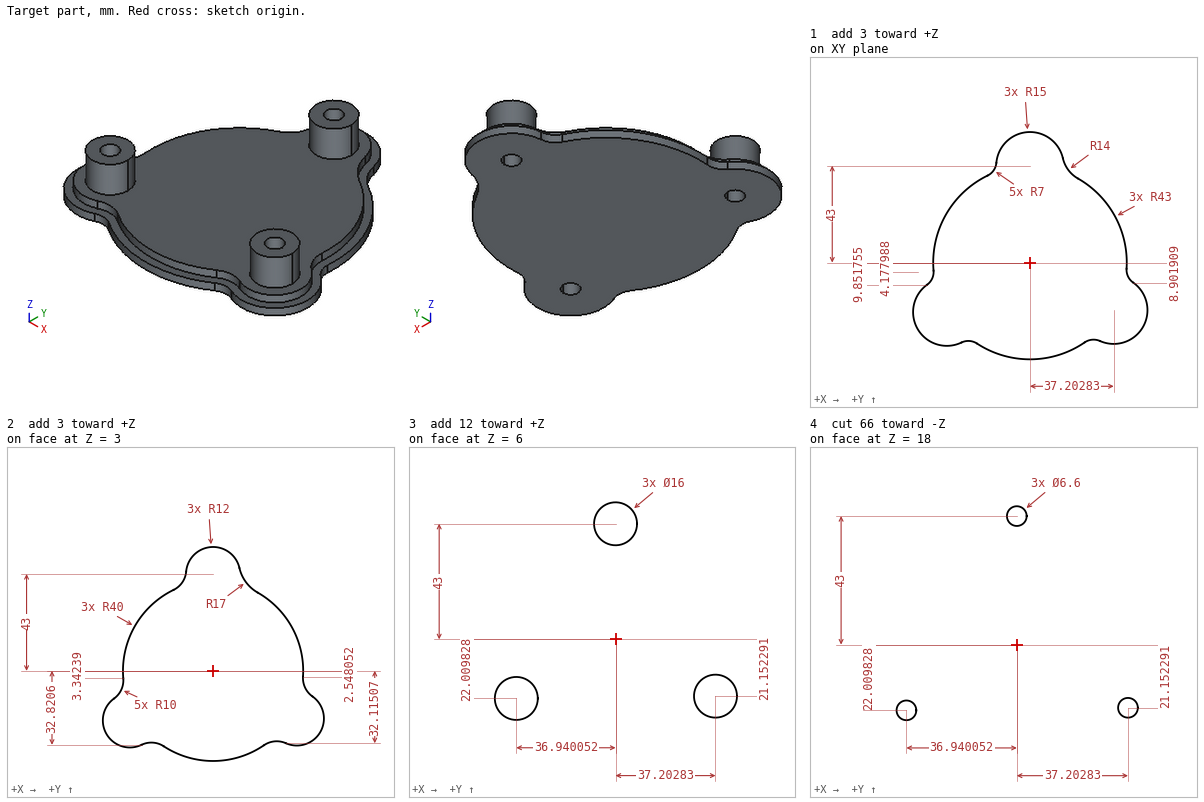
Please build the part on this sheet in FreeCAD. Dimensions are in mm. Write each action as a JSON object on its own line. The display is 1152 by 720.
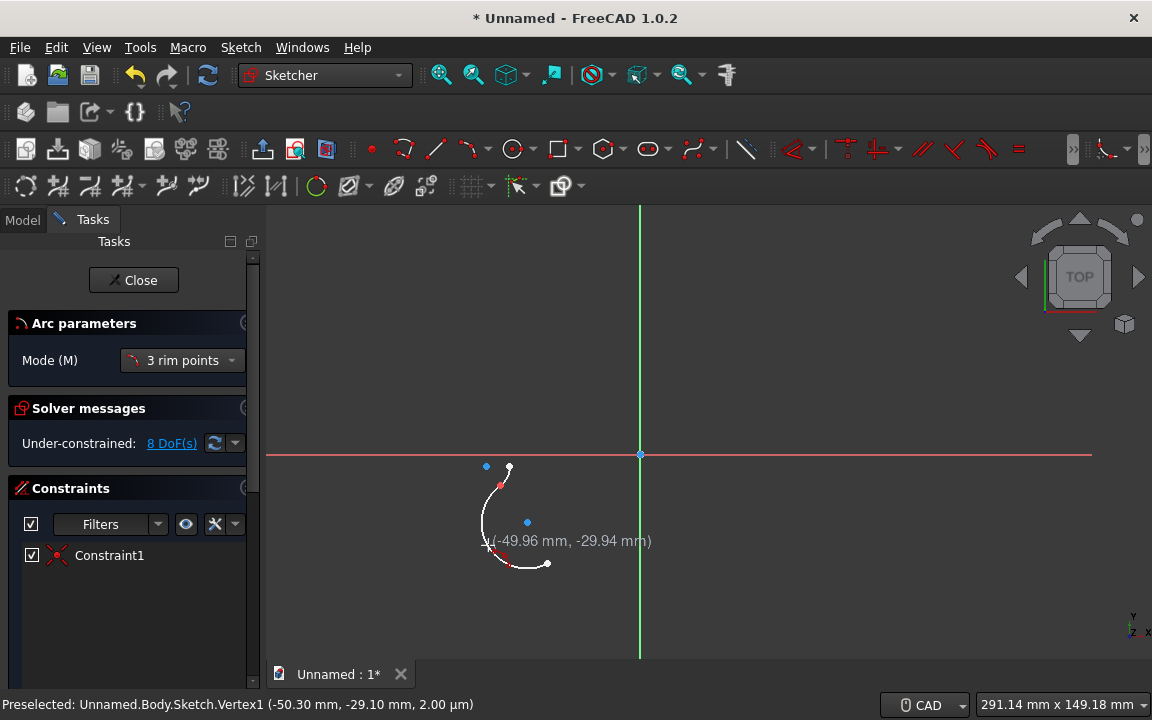
{"action": "left_click", "coordinate": [547, 564]}
{"action": "left_click", "coordinate": [568, 564]}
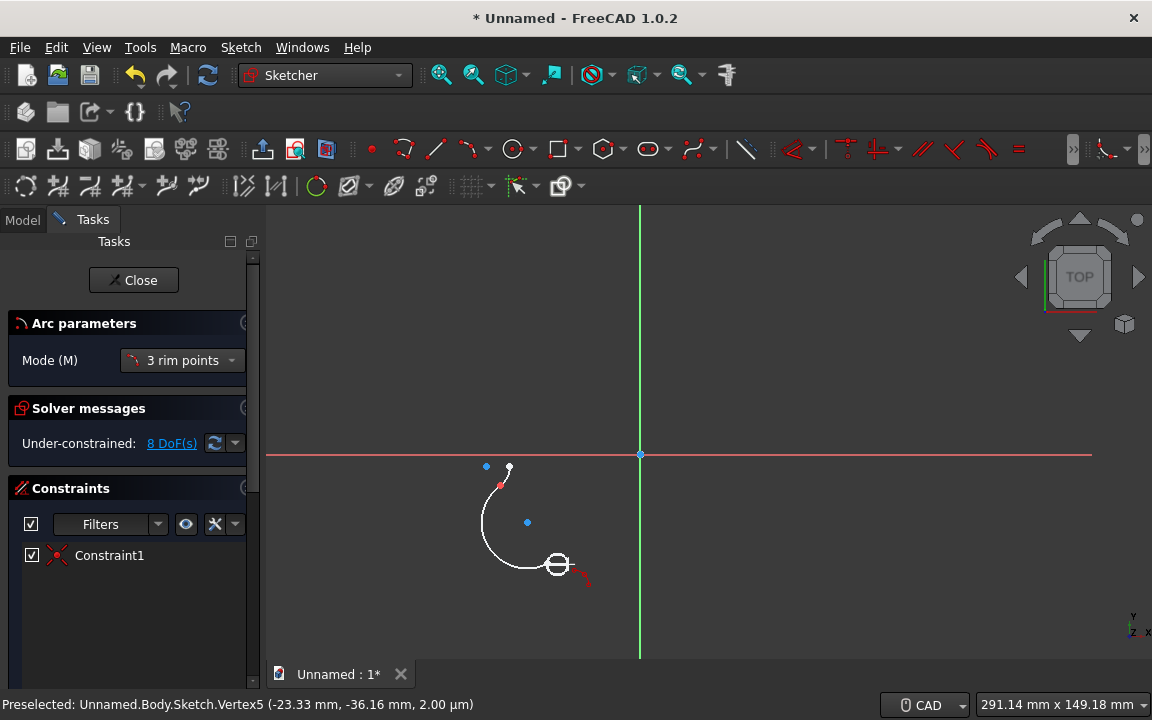
{"action": "scroll", "coordinate": [558, 561], "scroll_direction": "up", "scroll_amount": 9}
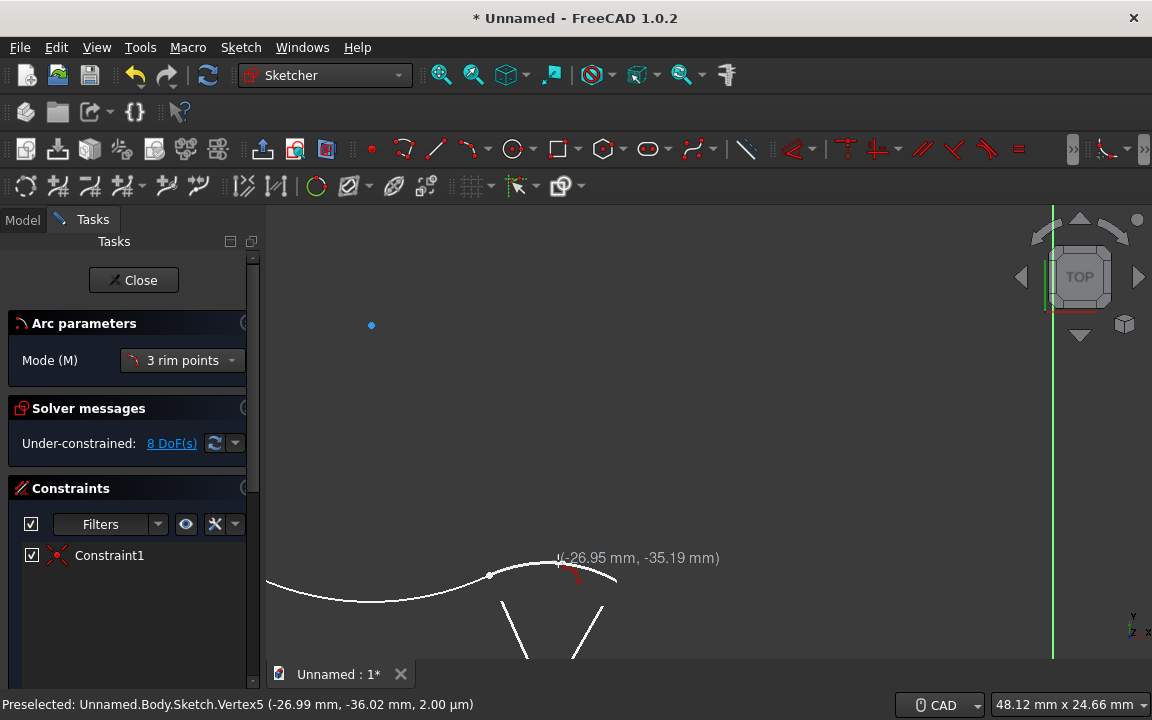
{"action": "left_click", "coordinate": [557, 557]}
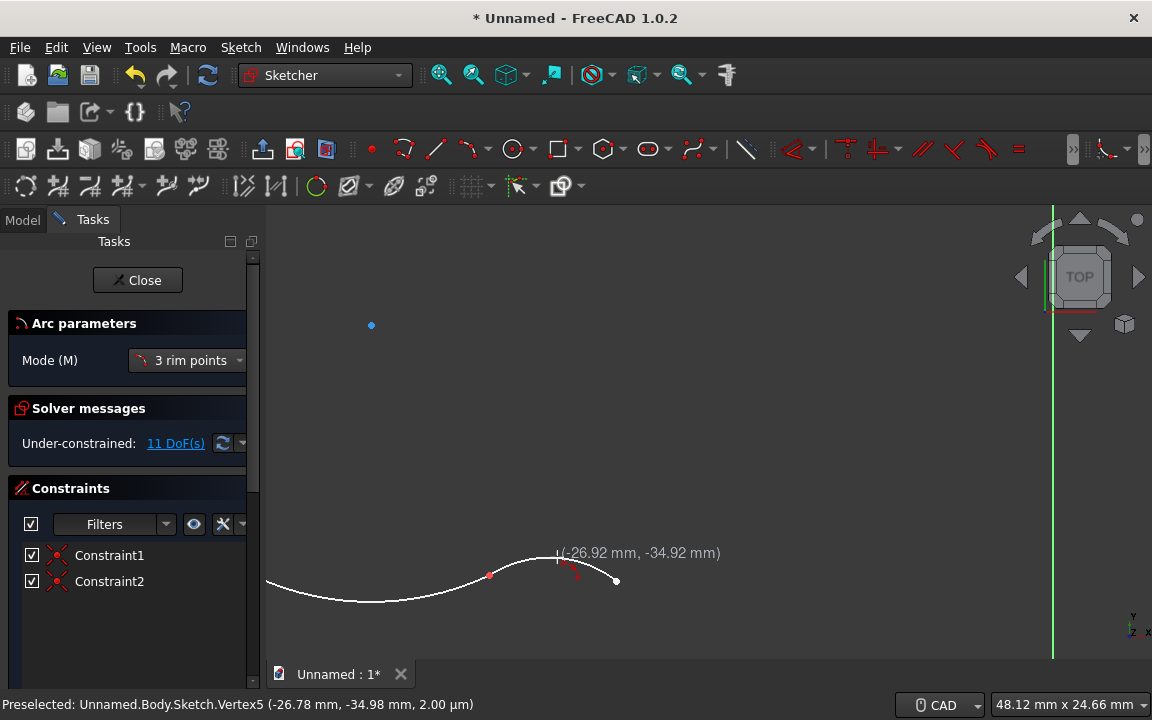
{"action": "scroll", "coordinate": [558, 562], "scroll_direction": "down", "scroll_amount": 9}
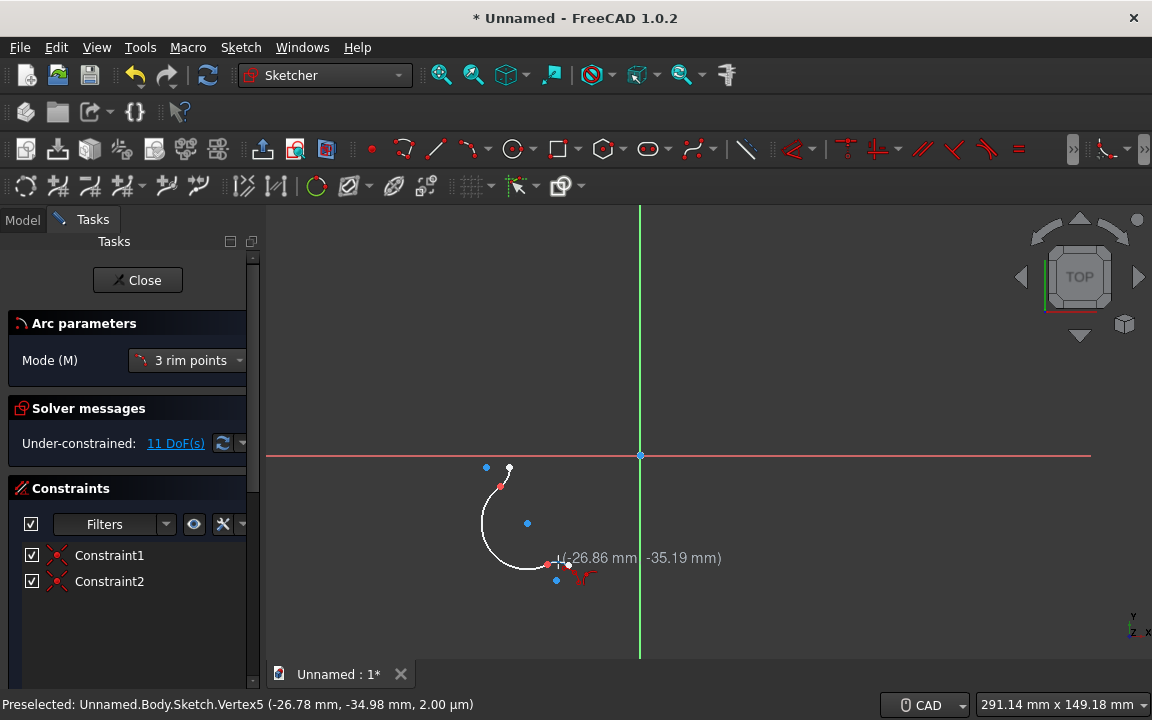
{"action": "left_click", "coordinate": [568, 566]}
{"action": "left_click", "coordinate": [714, 564]}
{"action": "left_click", "coordinate": [626, 586]}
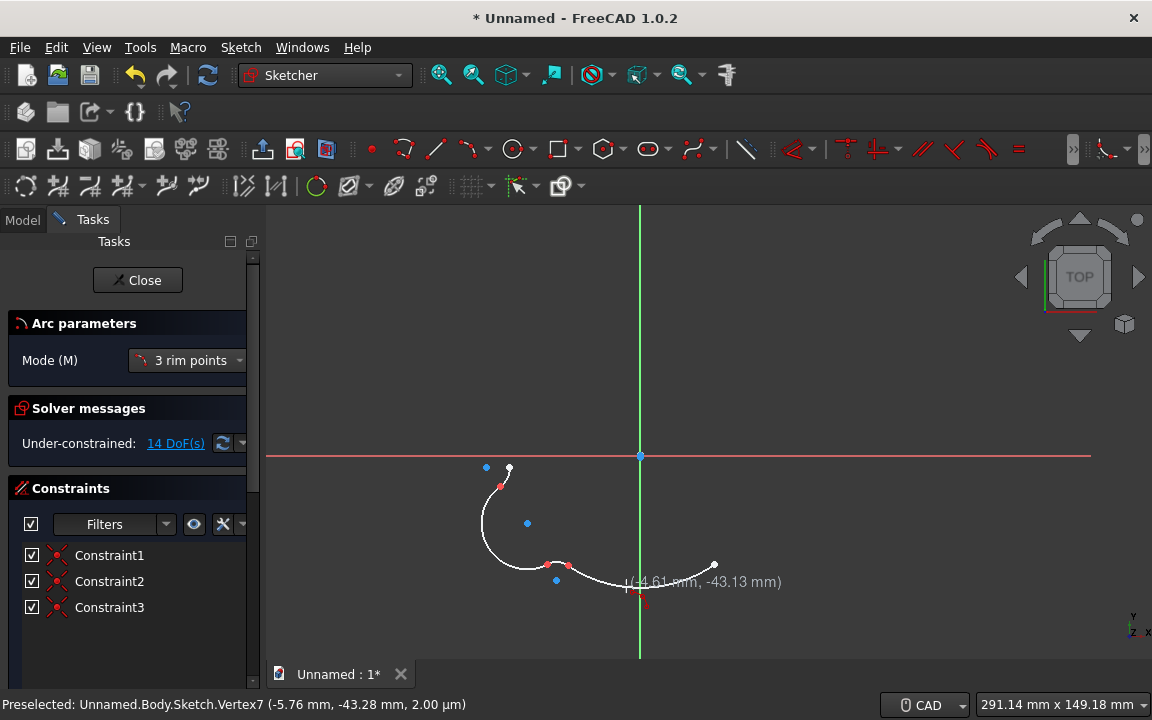
{"action": "left_click", "coordinate": [714, 565]}
{"action": "left_click", "coordinate": [735, 562]}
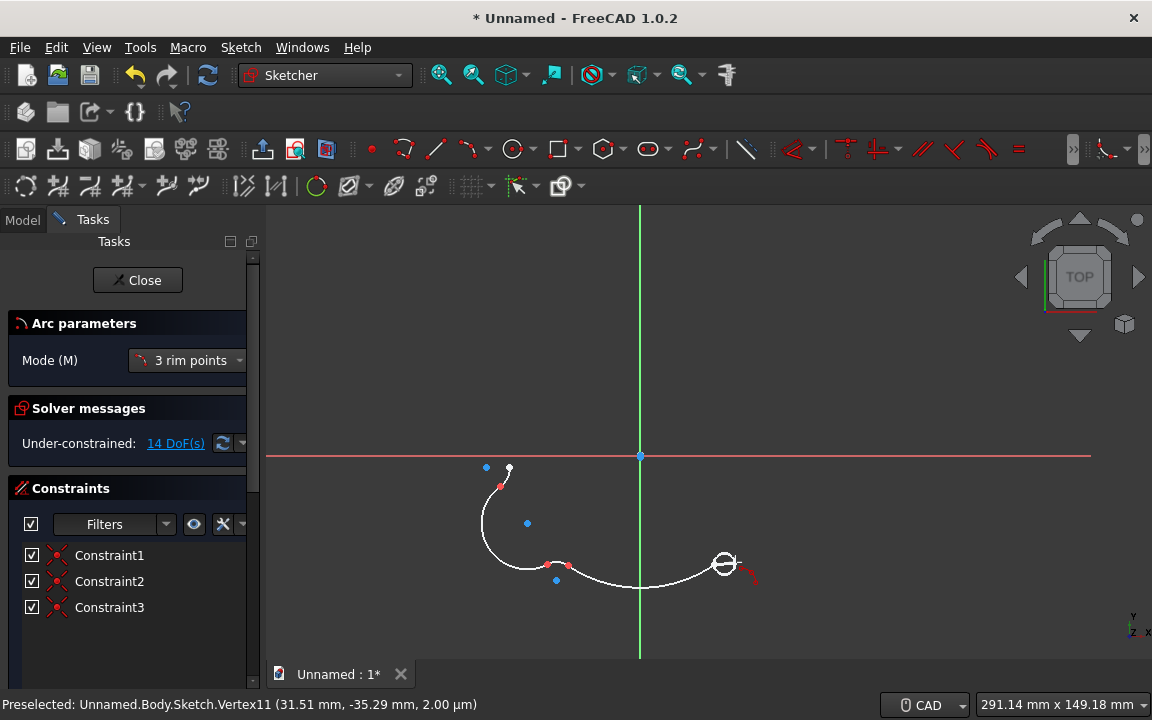
{"action": "scroll", "coordinate": [724, 560], "scroll_direction": "up", "scroll_amount": 9}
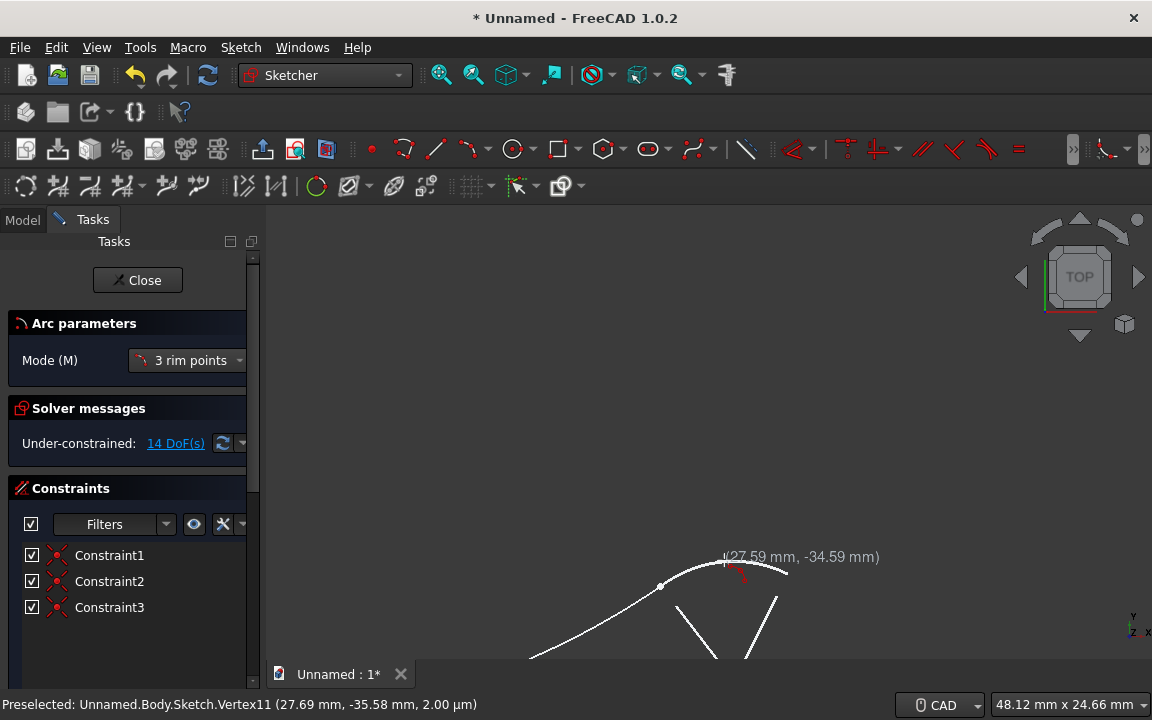
{"action": "left_click", "coordinate": [722, 556]}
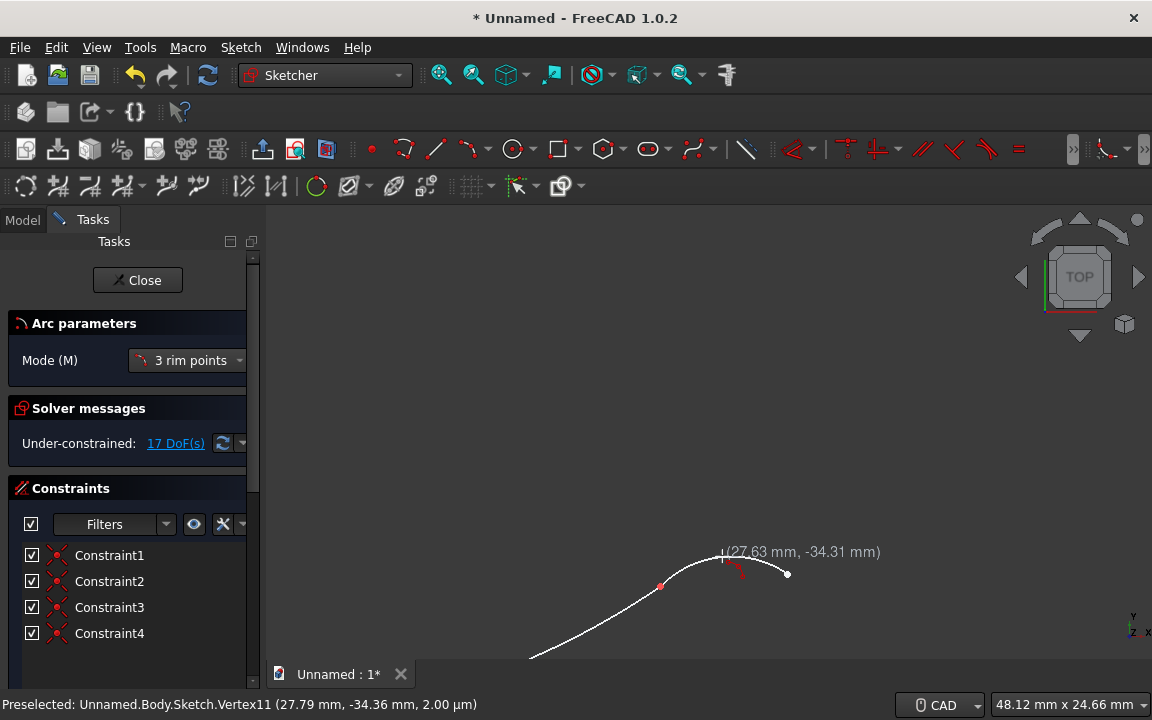
{"action": "scroll", "coordinate": [724, 560], "scroll_direction": "down", "scroll_amount": 9}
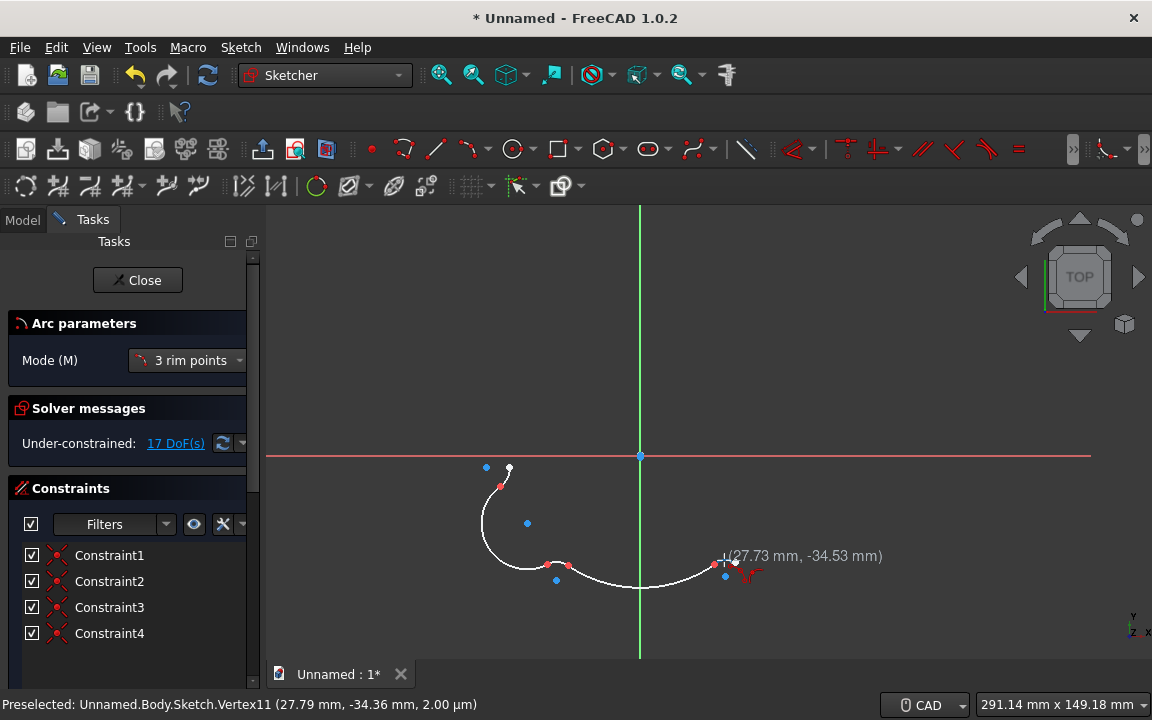
{"action": "left_click", "coordinate": [735, 563]}
{"action": "left_click", "coordinate": [780, 483]}
{"action": "left_click", "coordinate": [793, 543]}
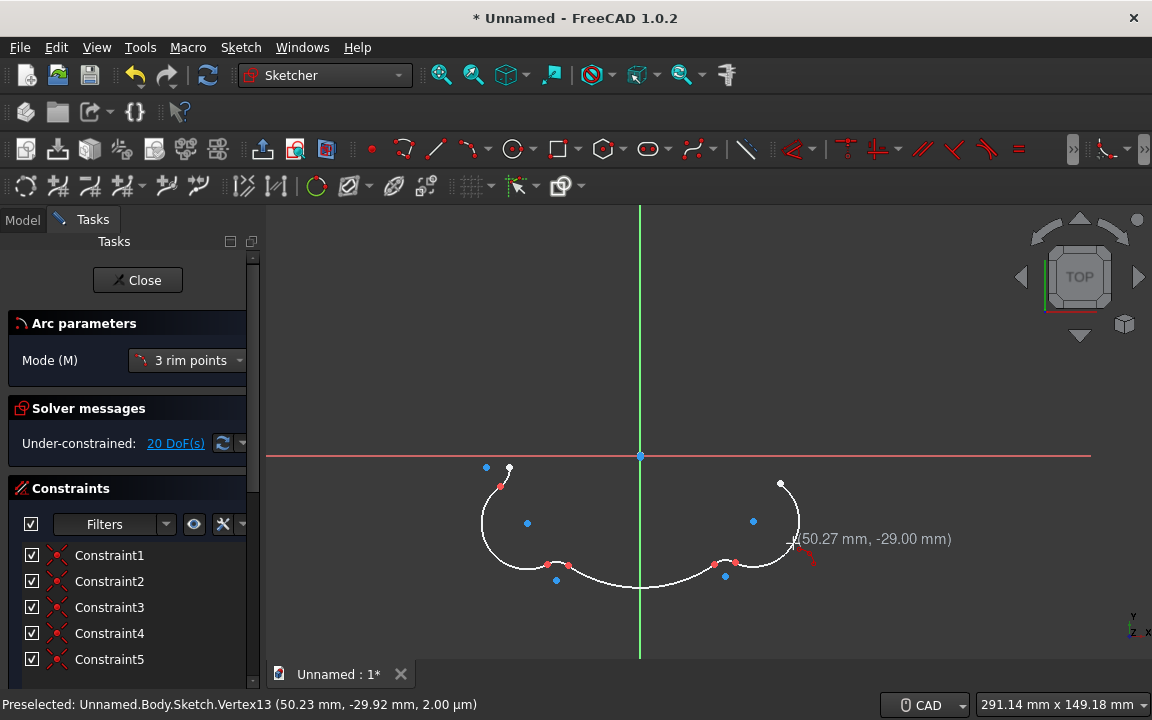
{"action": "left_click", "coordinate": [780, 484]}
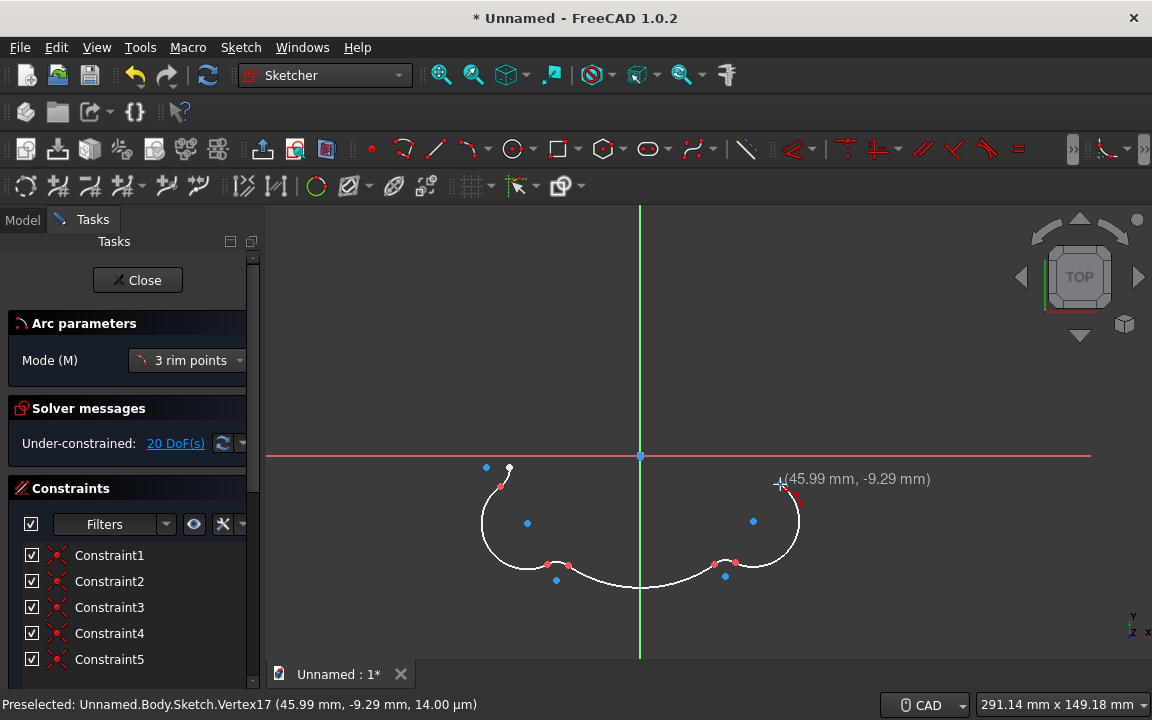
{"action": "scroll", "coordinate": [771, 464], "scroll_direction": "up", "scroll_amount": 4}